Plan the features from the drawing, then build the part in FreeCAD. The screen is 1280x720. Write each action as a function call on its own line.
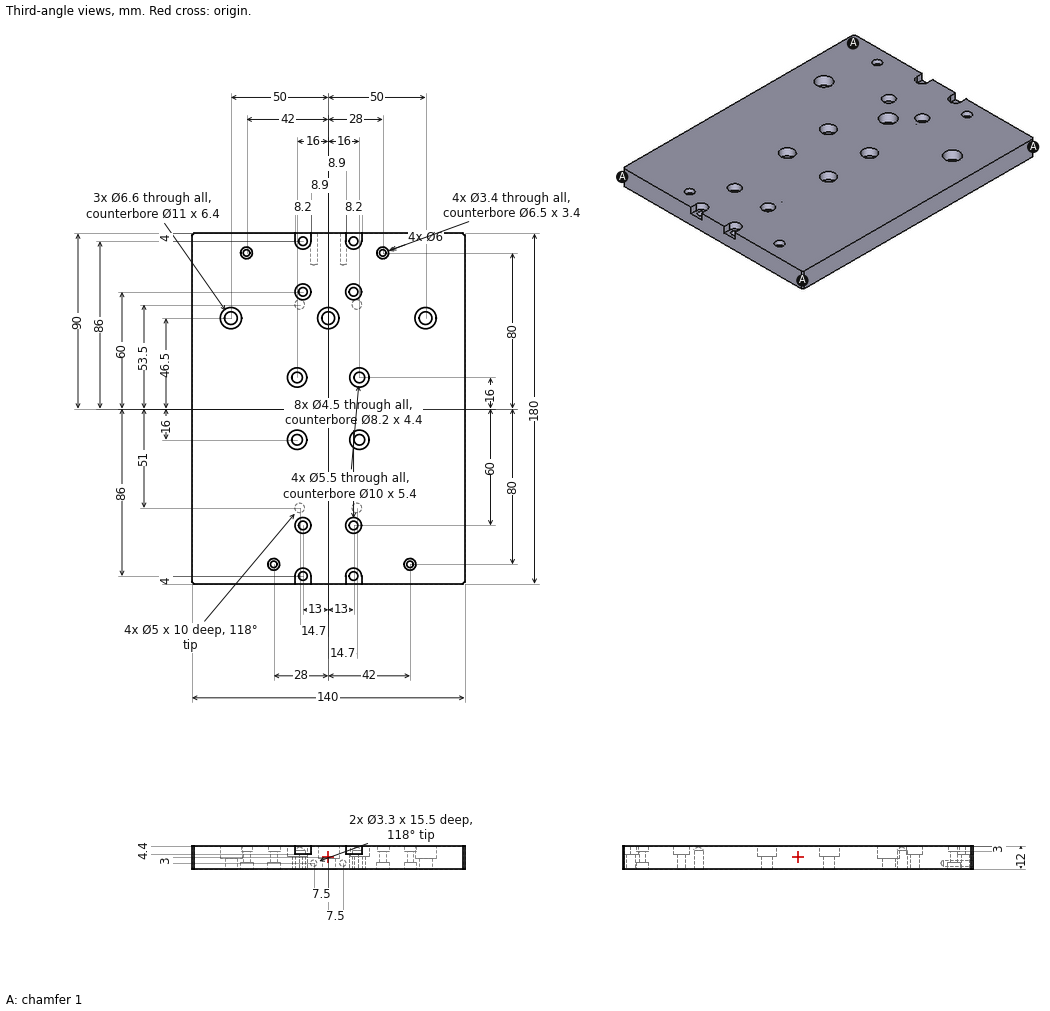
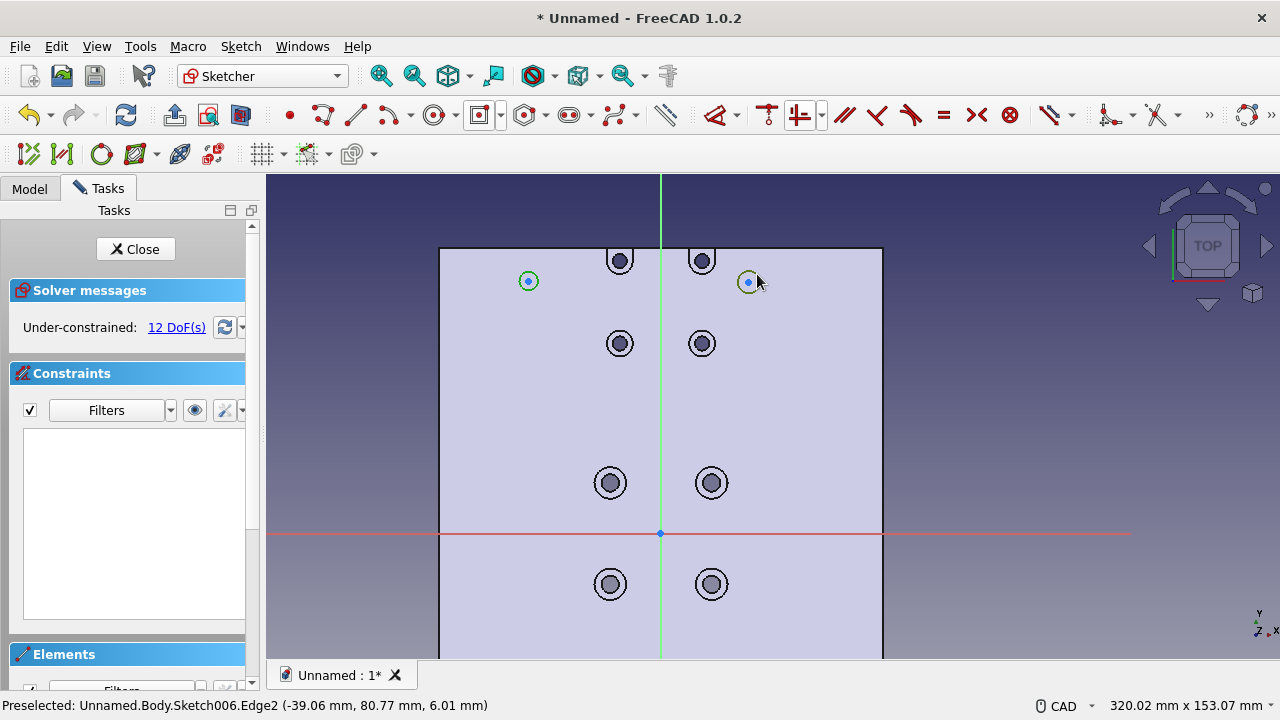
scroll(782, 553, up, 5)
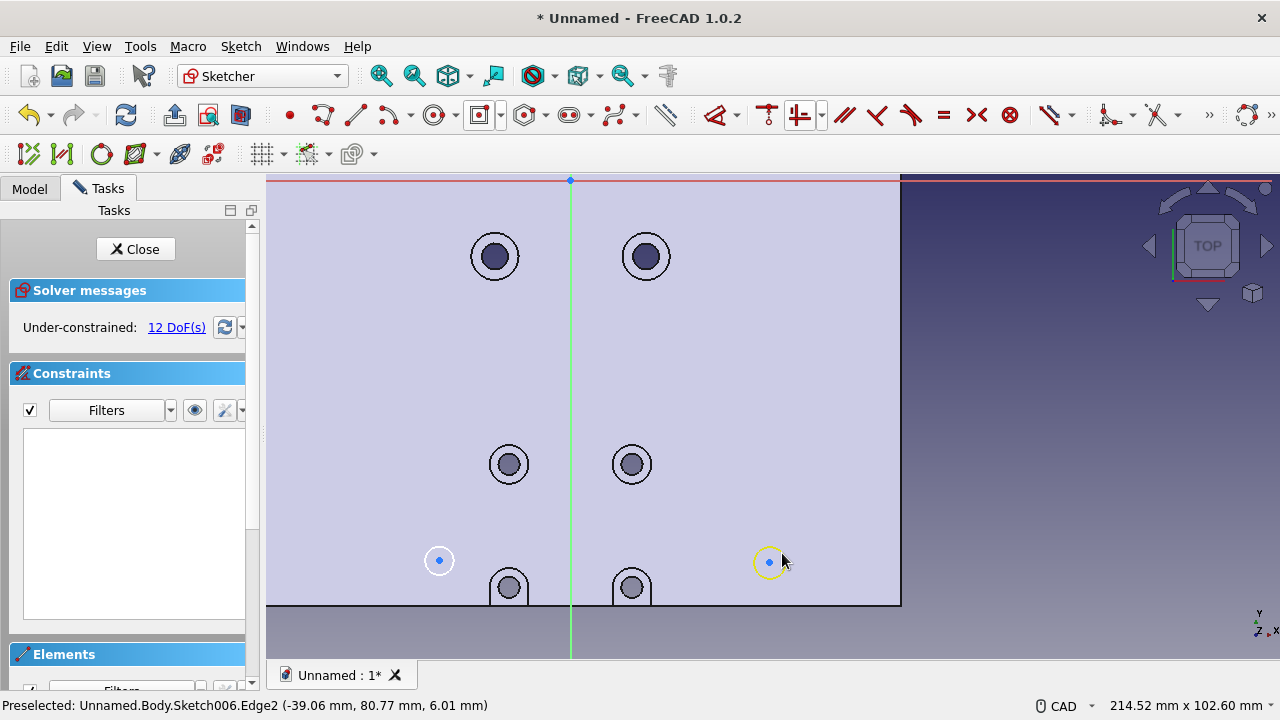
click(781, 552)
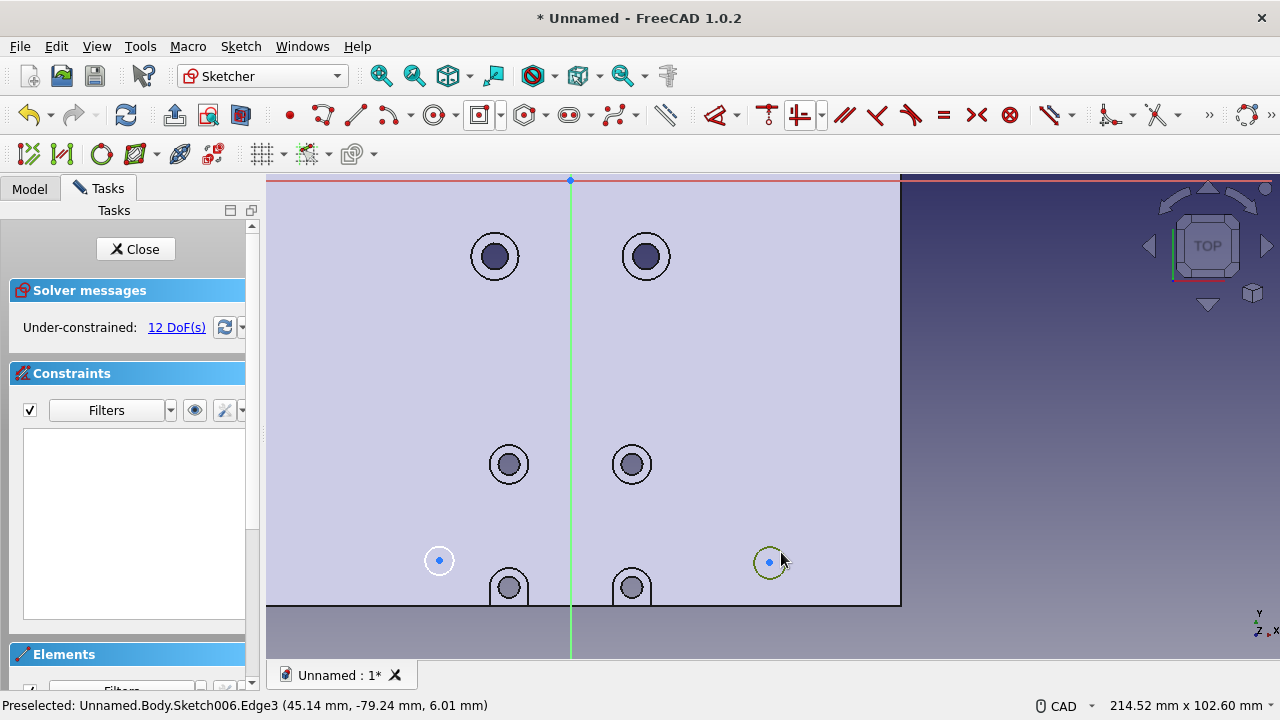
click(449, 551)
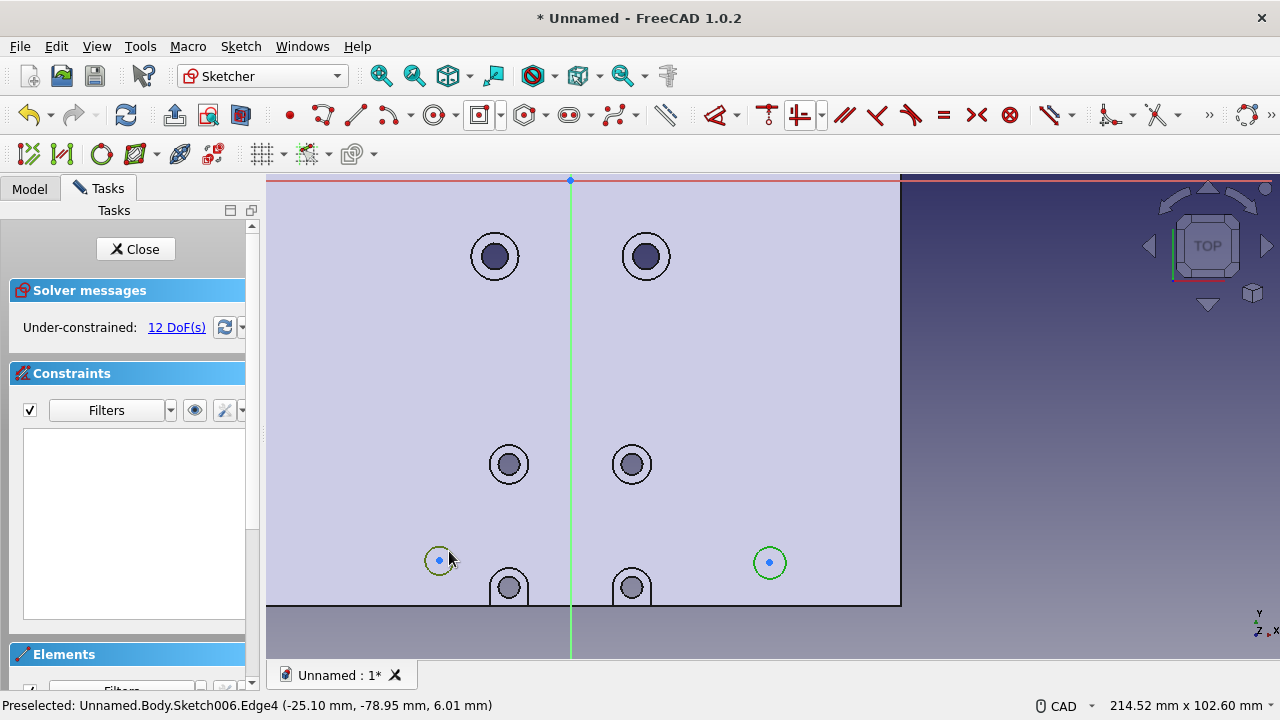
click(944, 116)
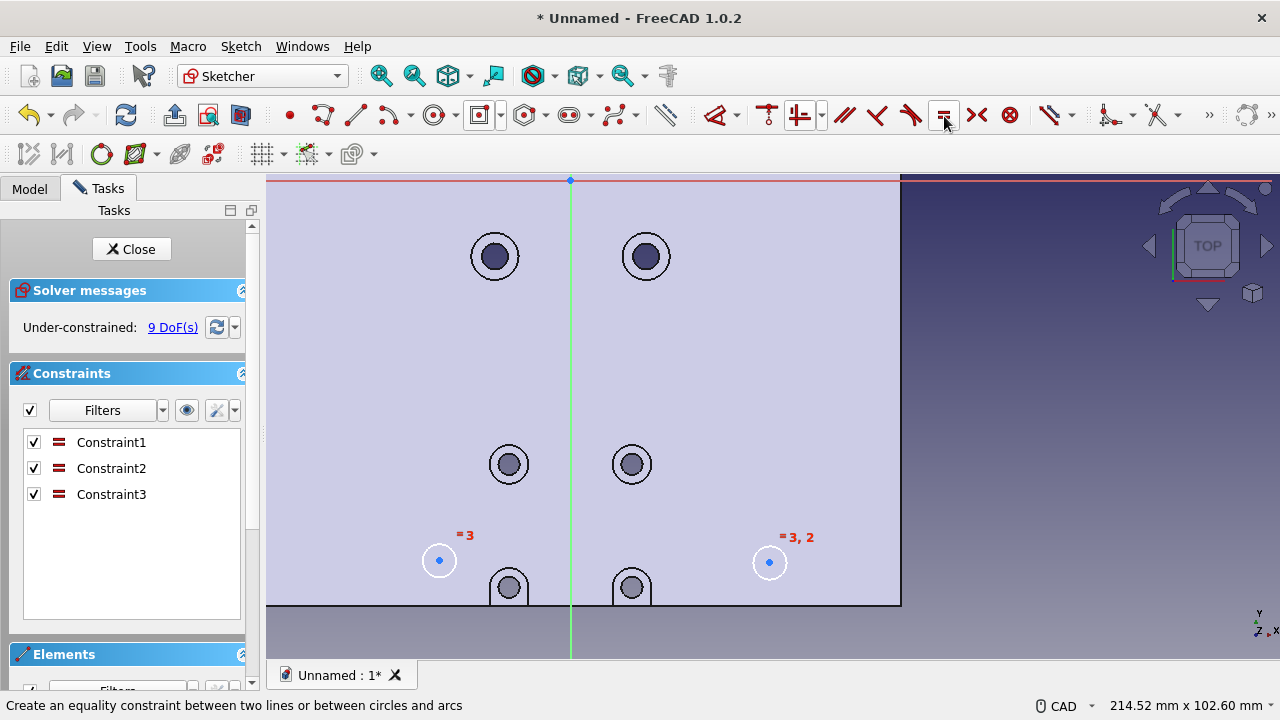
click(714, 116)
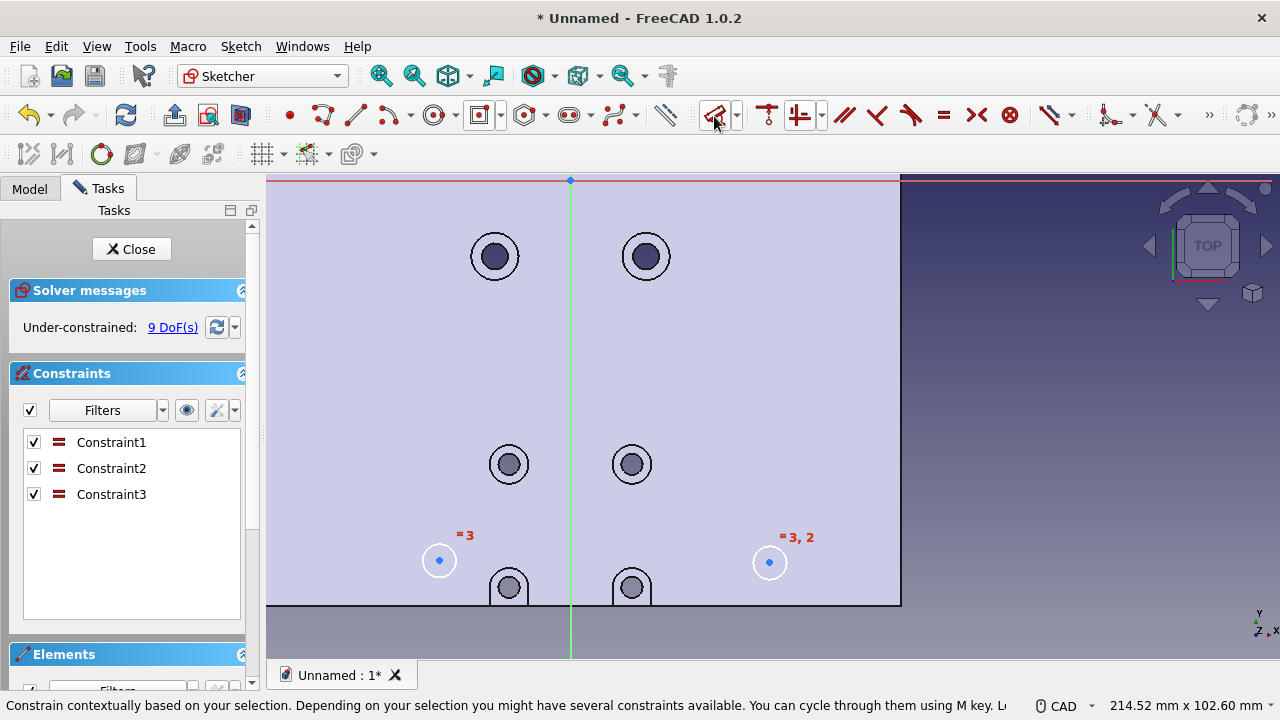
scroll(782, 554, down, 5)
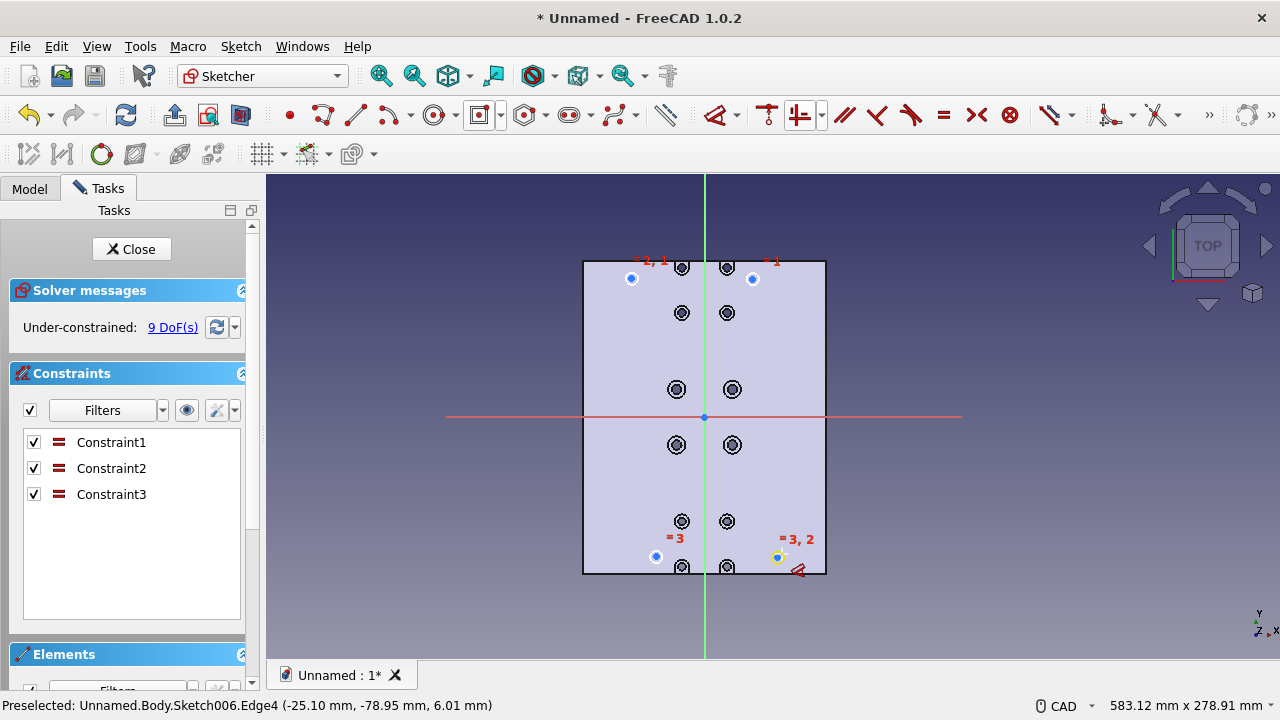
scroll(757, 275, up, 7)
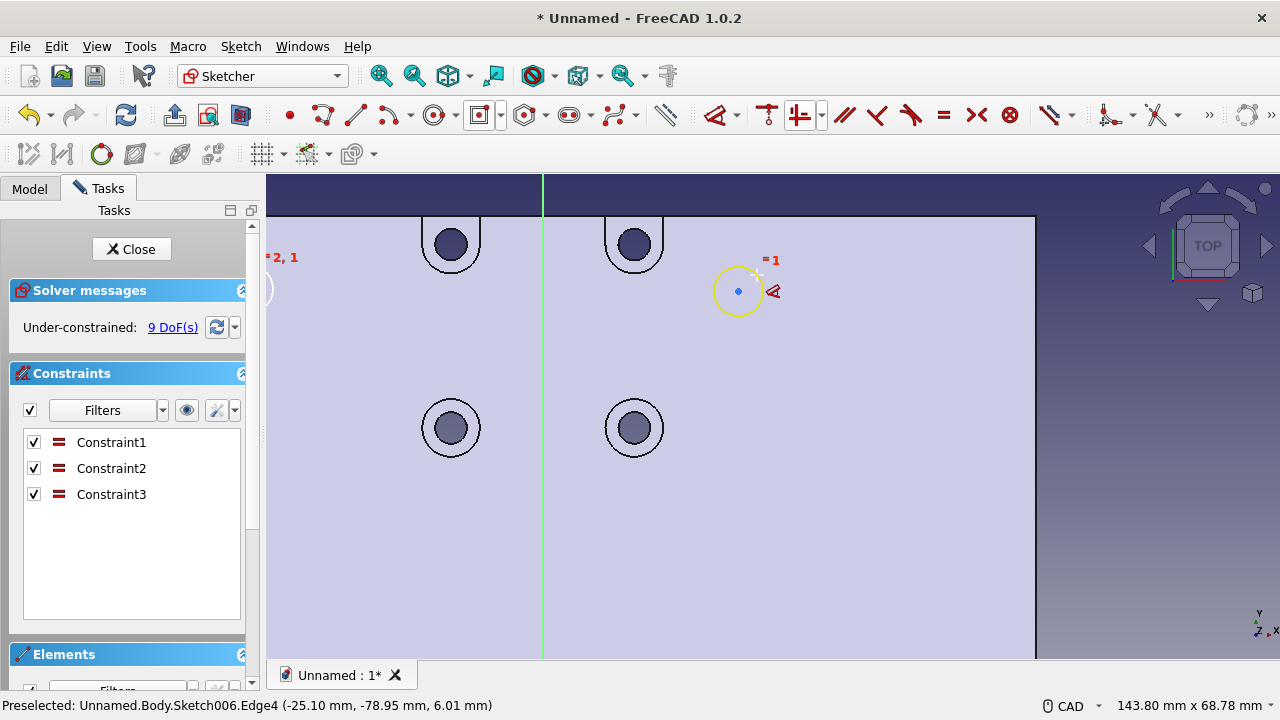
click(756, 274)
click(779, 251)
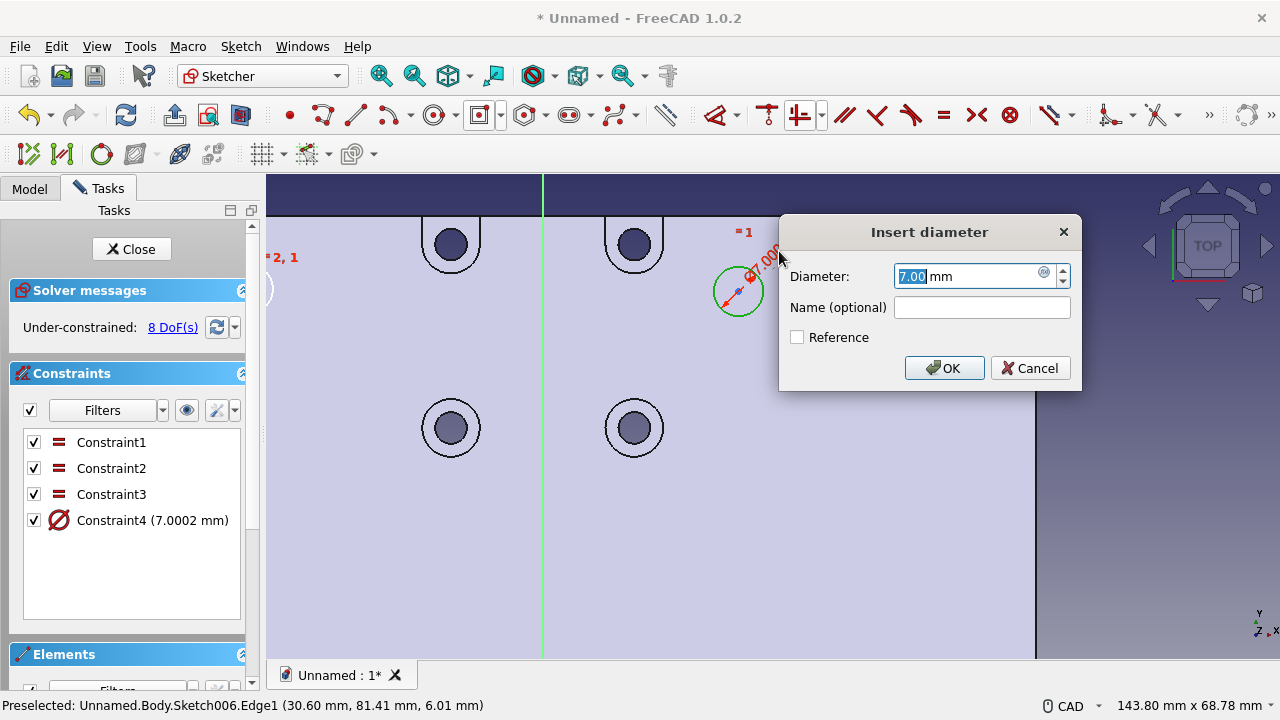
text(6)
key(Return)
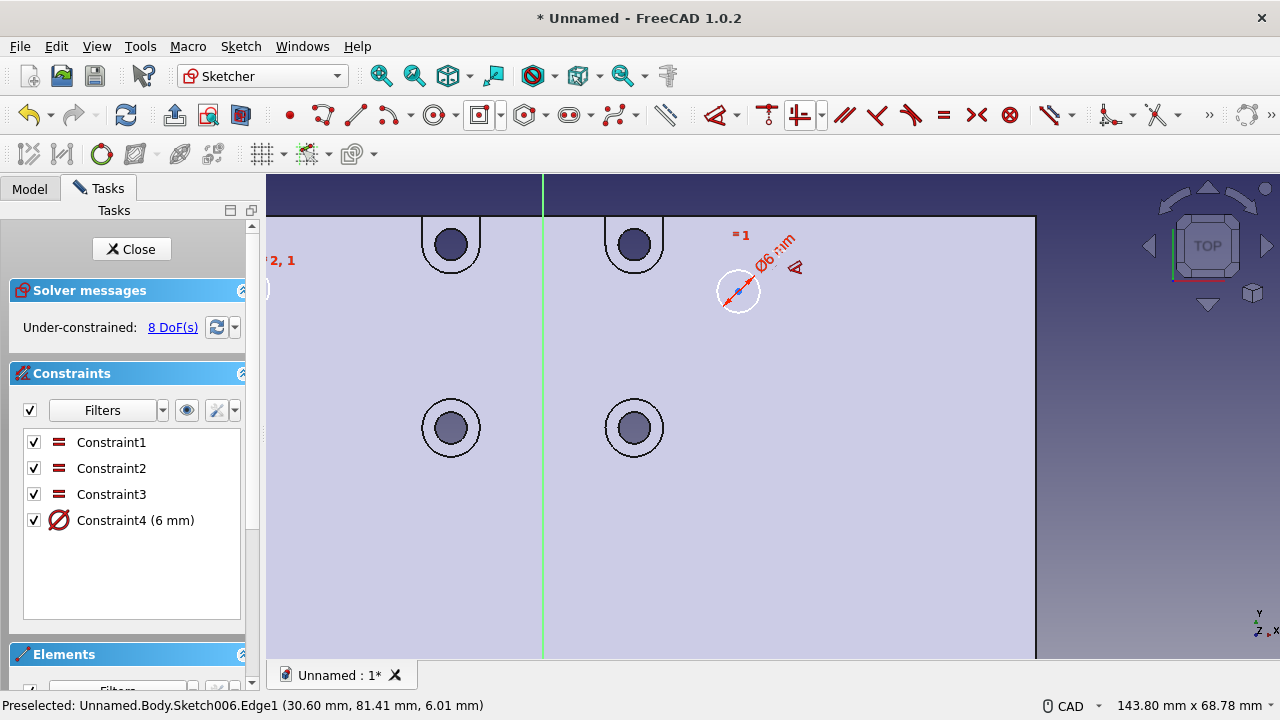
click(739, 291)
click(641, 257)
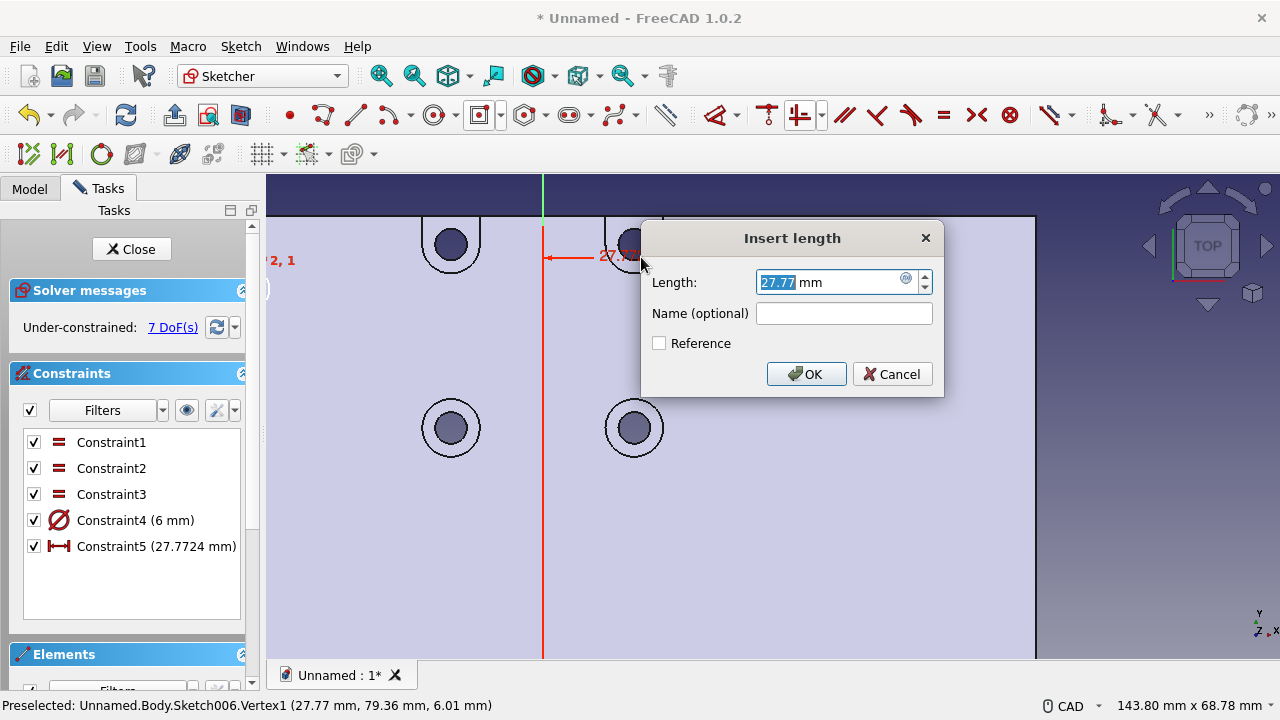
text(28)
key(Return)